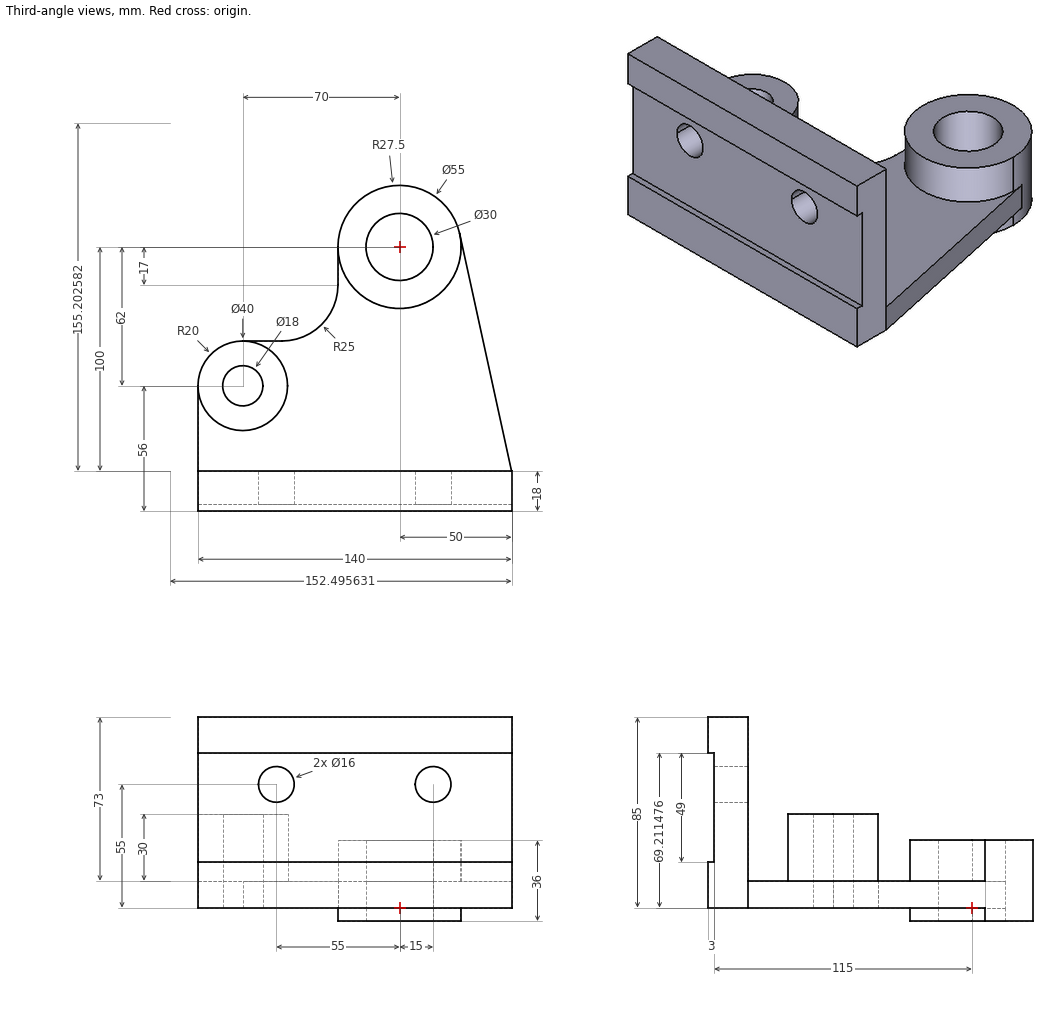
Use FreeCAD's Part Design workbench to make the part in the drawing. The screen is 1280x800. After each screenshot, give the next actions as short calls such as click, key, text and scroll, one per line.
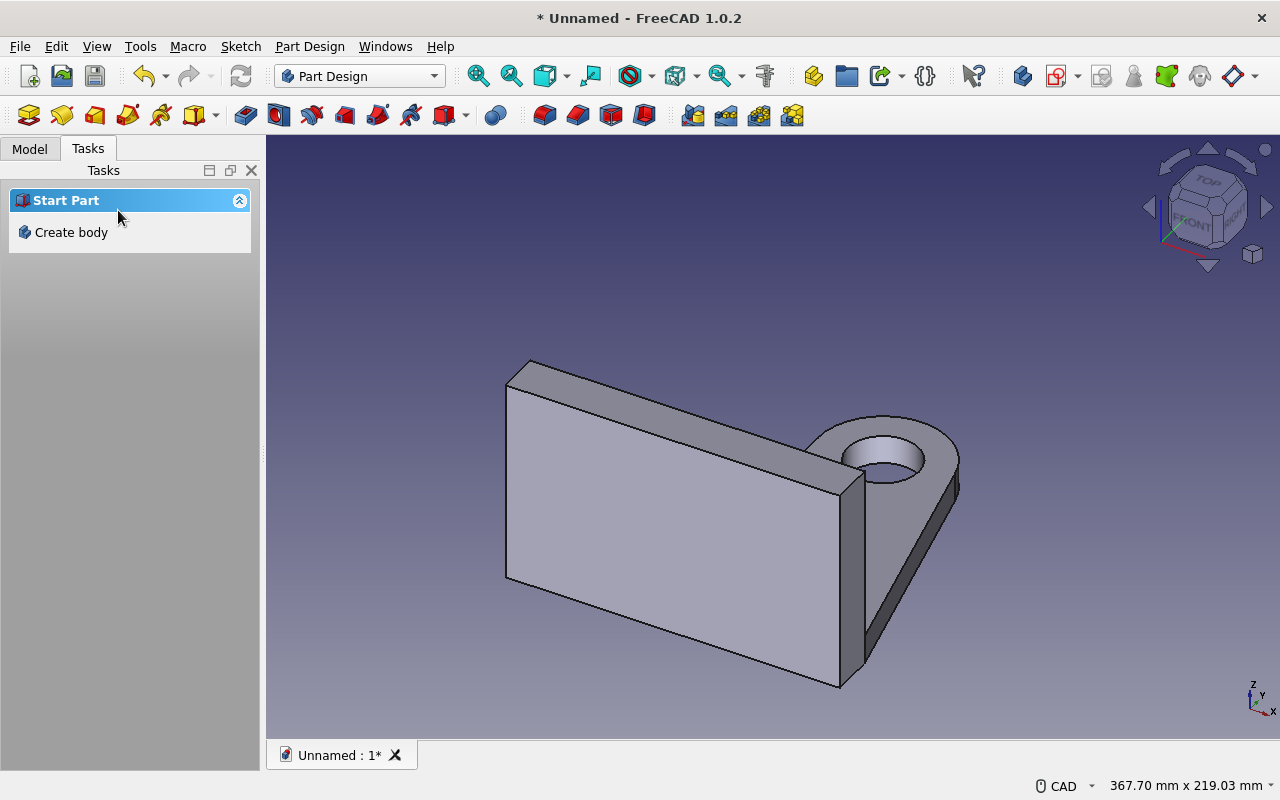
key(6)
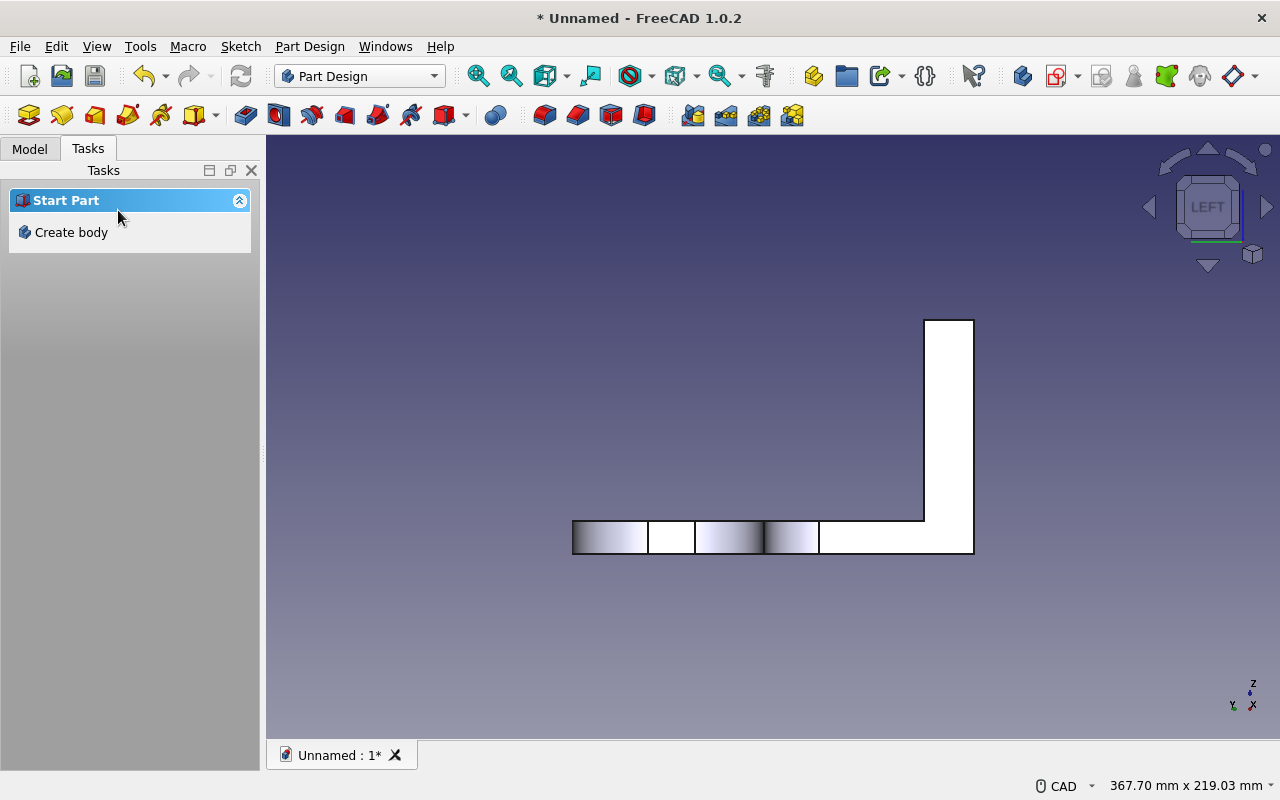
click(479, 76)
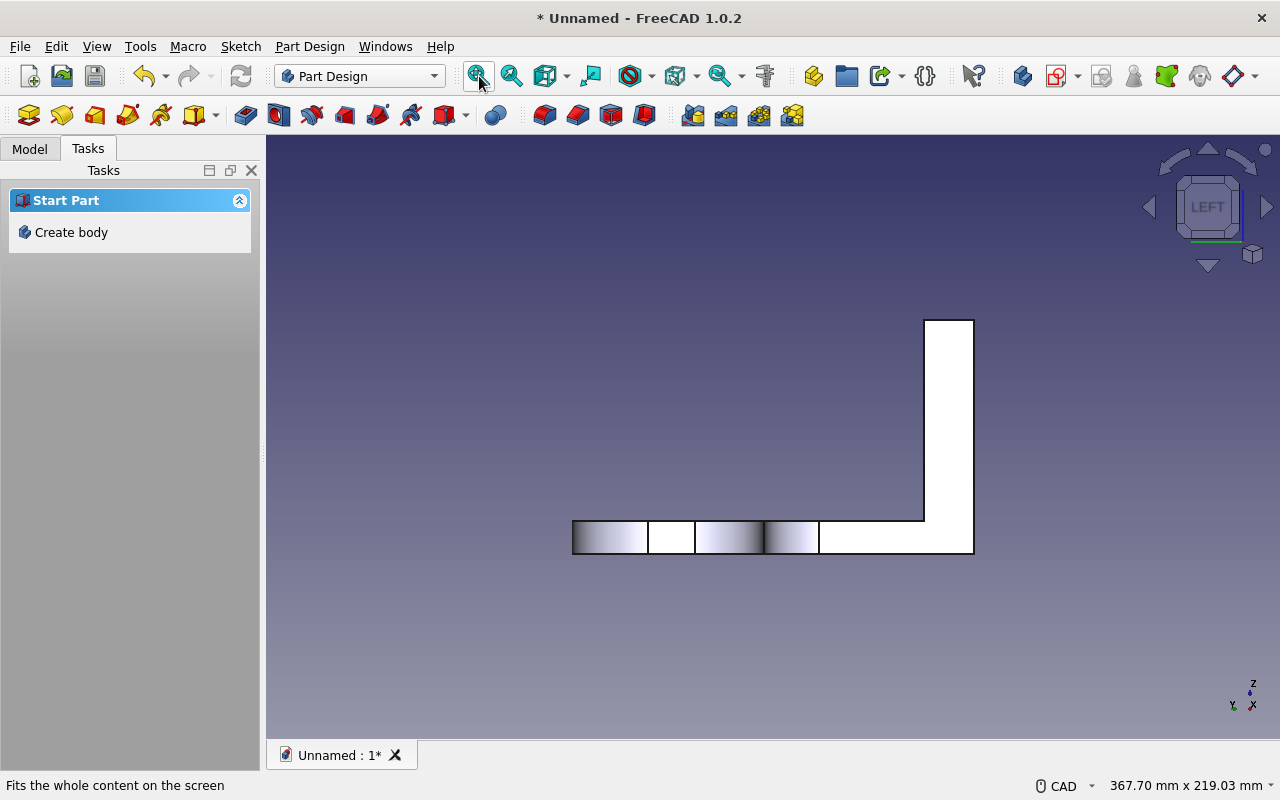
click(940, 536)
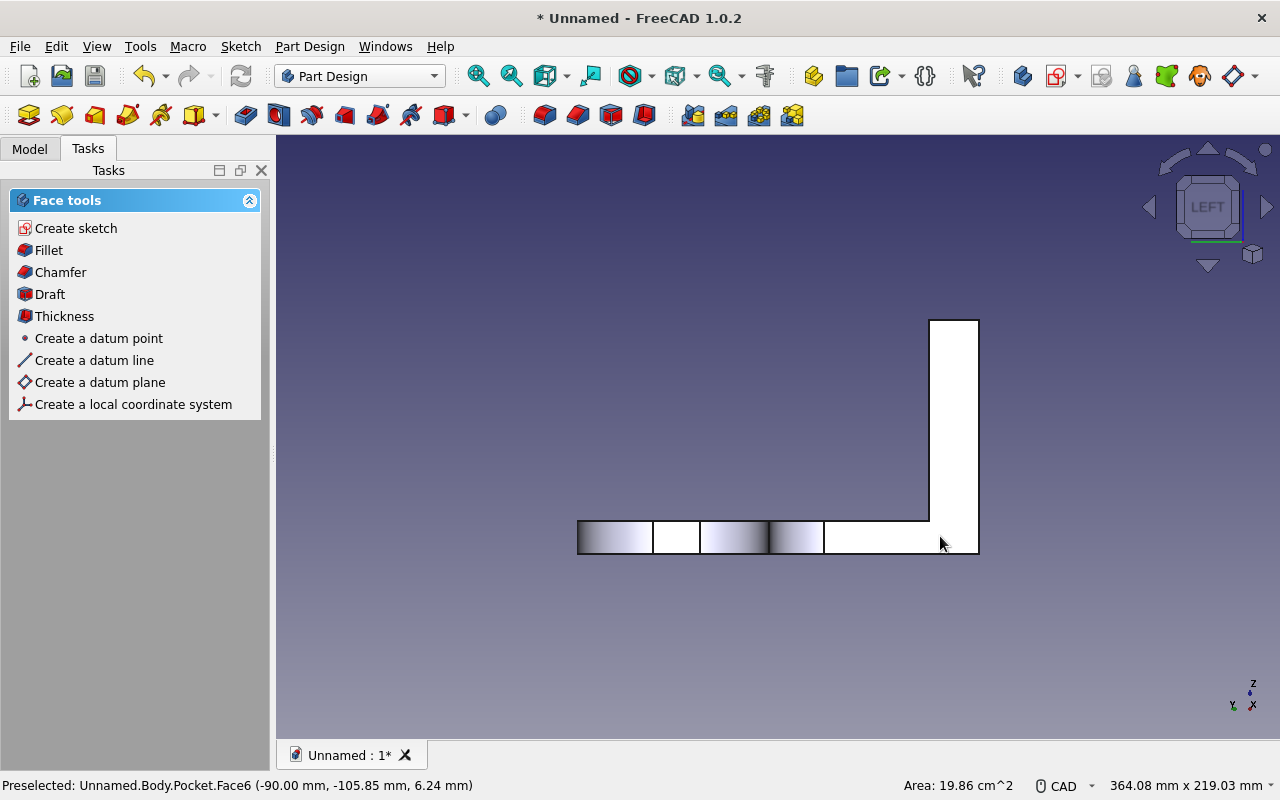
click(1056, 76)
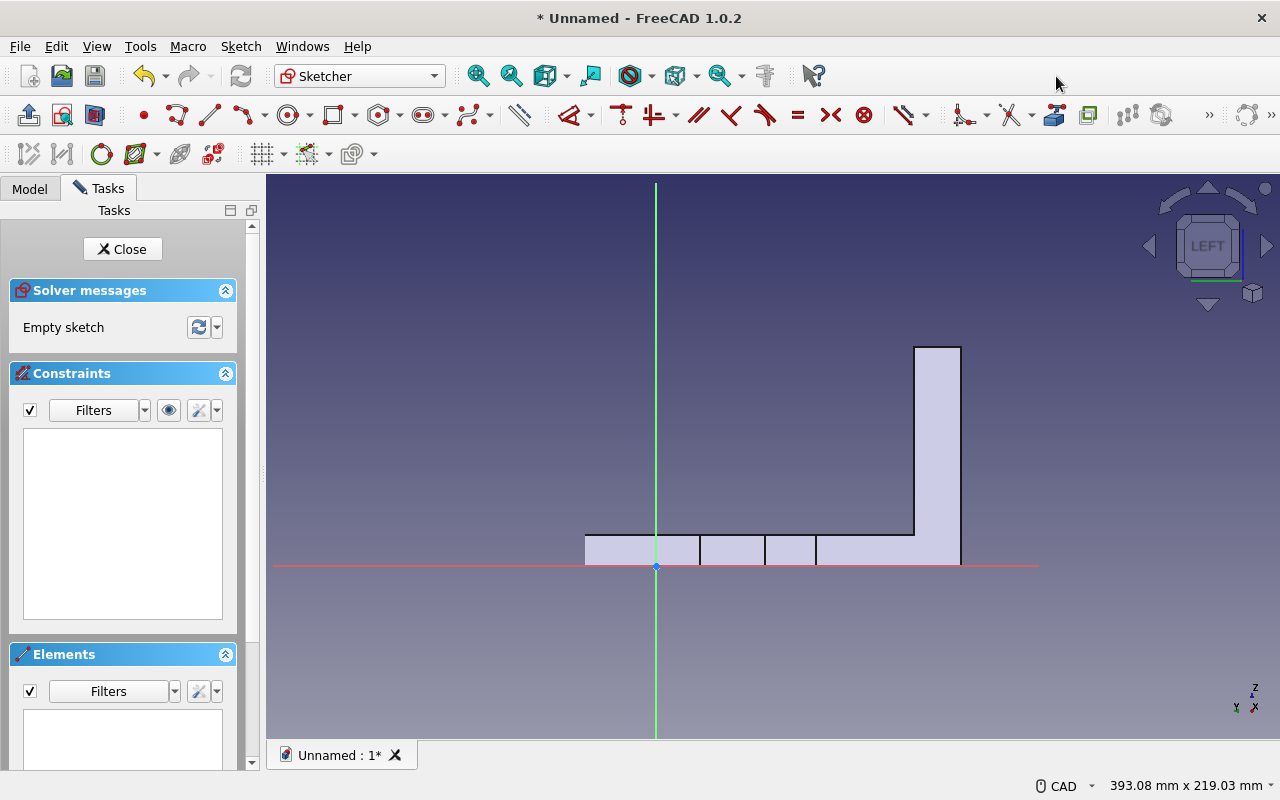
scroll(935, 502, up, 3)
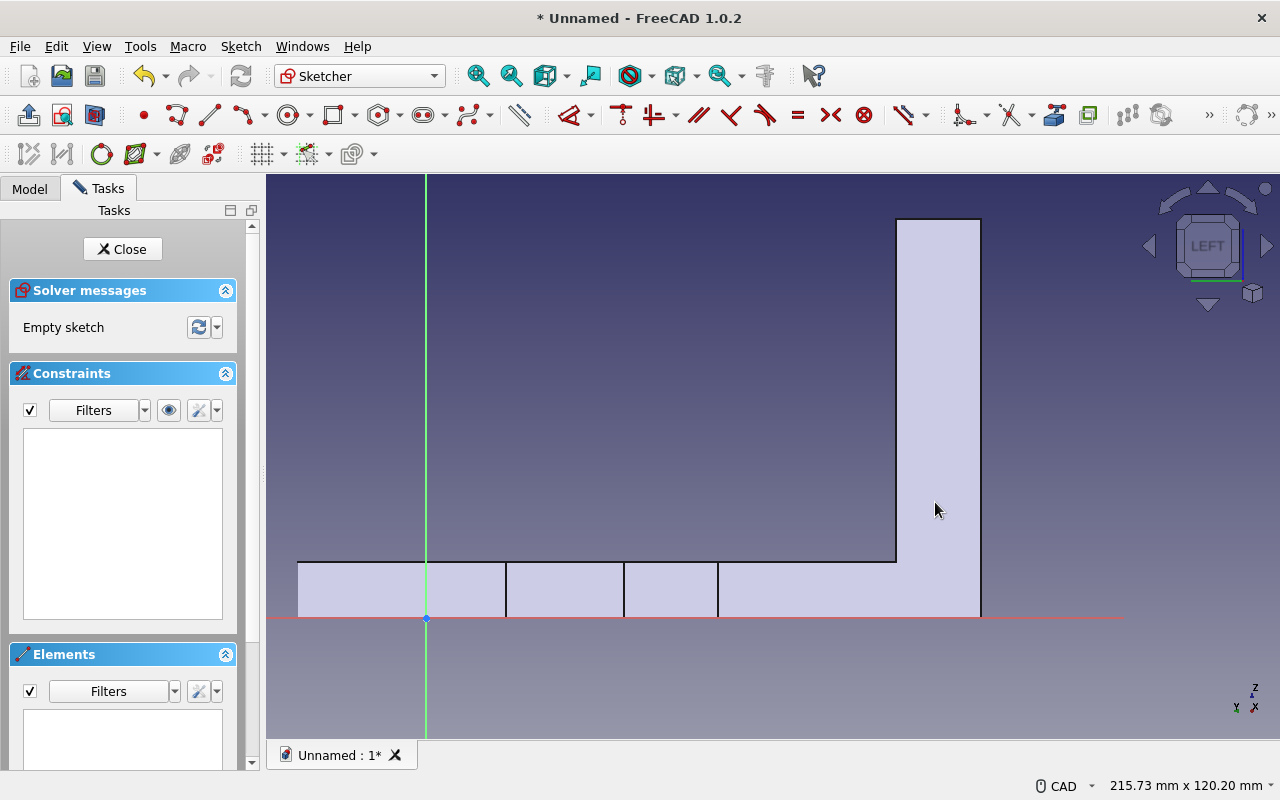
key(g)
key(r)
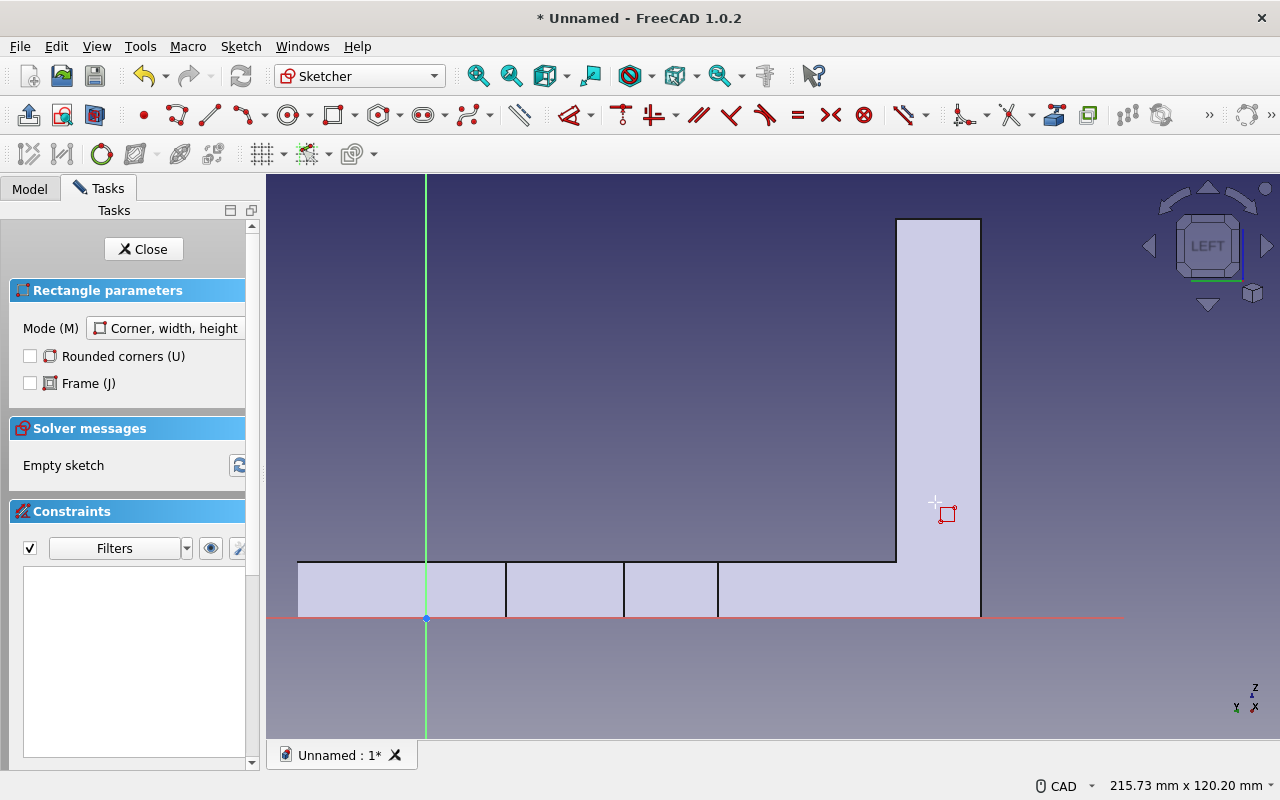
click(967, 293)
click(981, 523)
key(Escape)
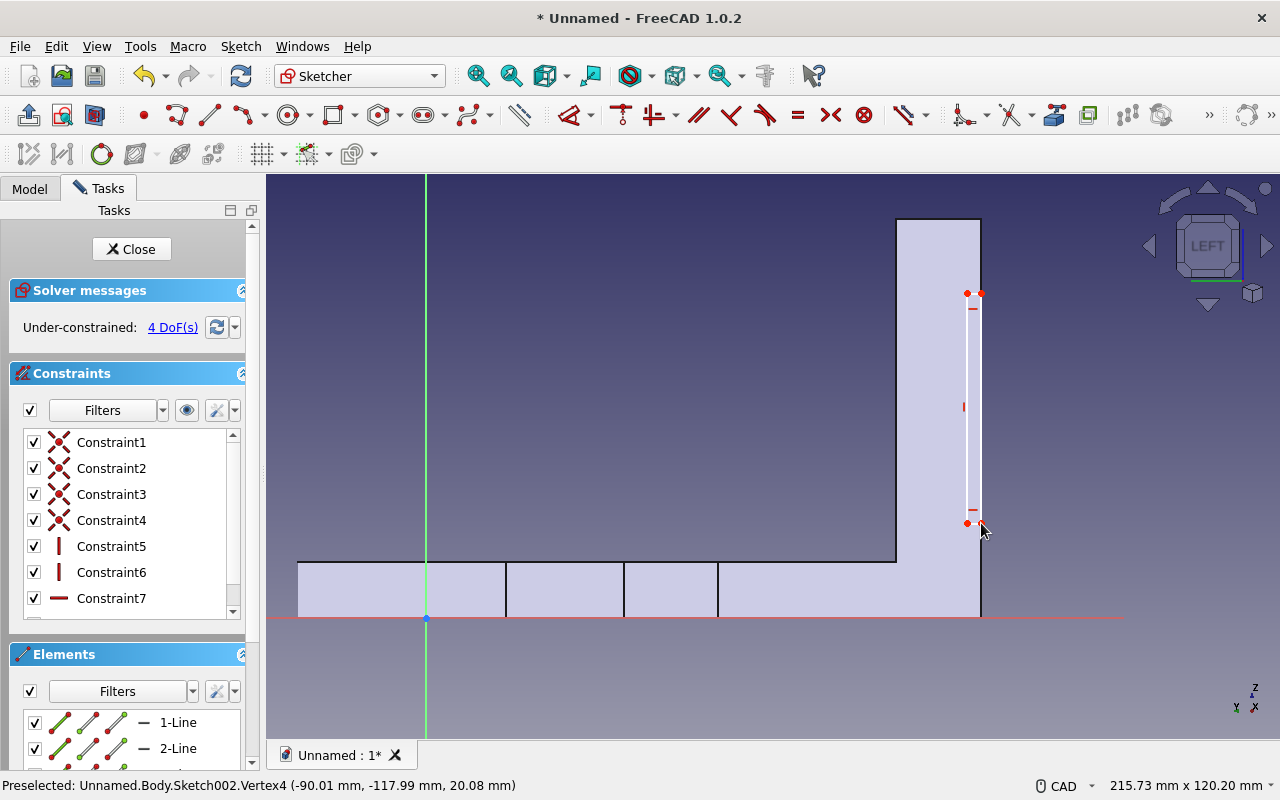
click(568, 116)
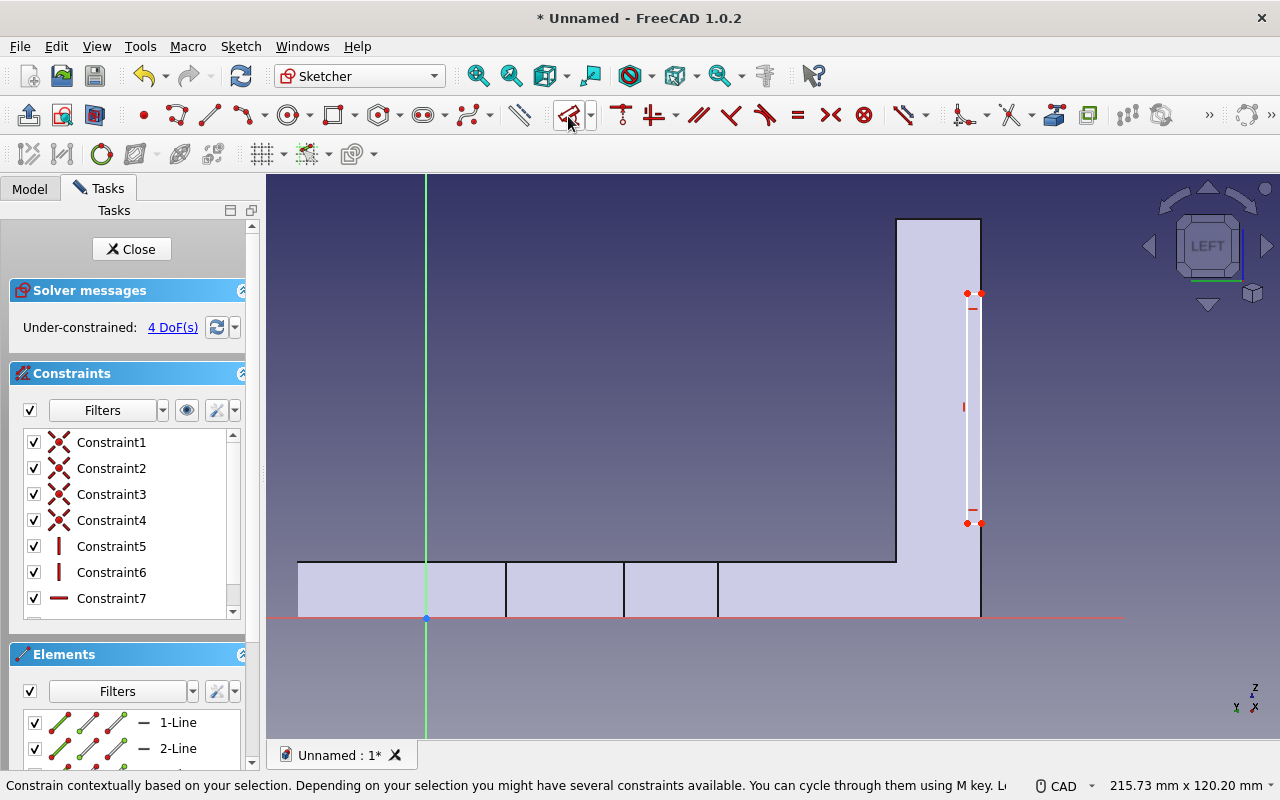
scroll(974, 524, up, 6)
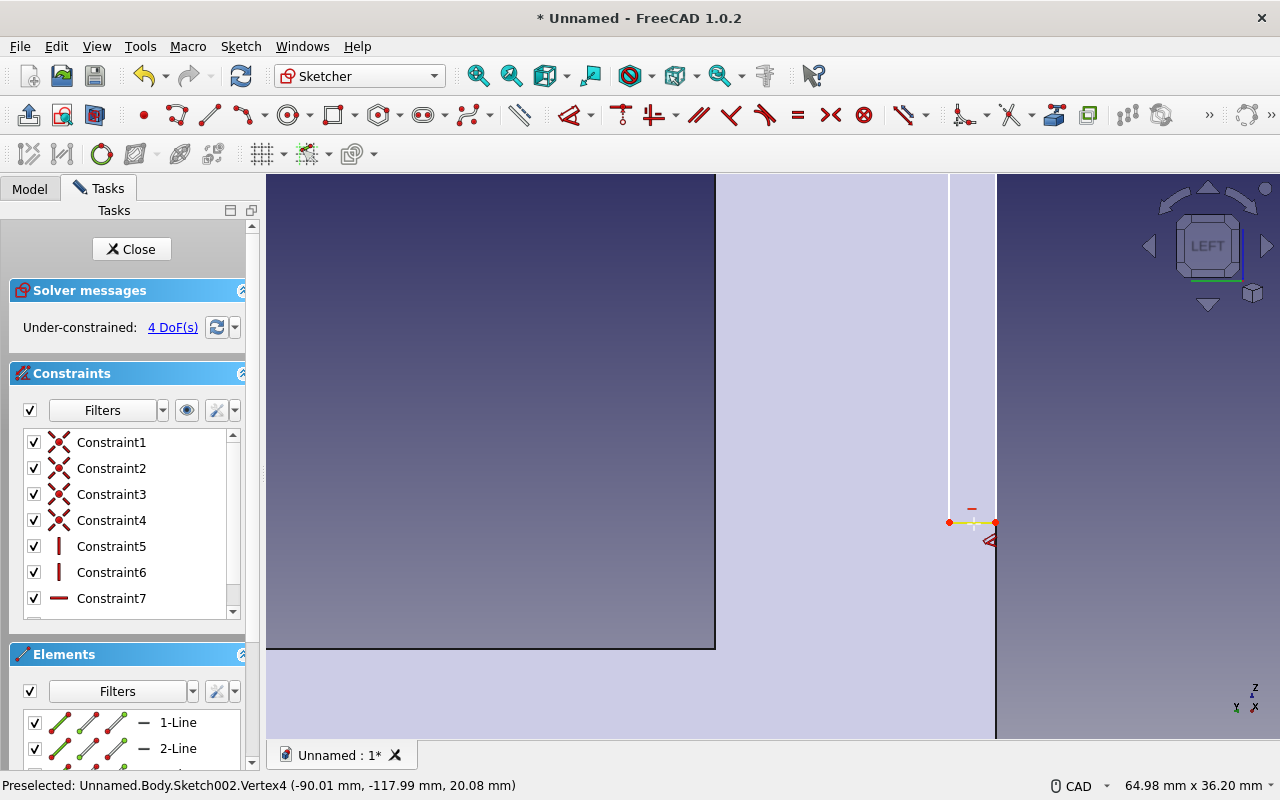
click(972, 523)
click(972, 557)